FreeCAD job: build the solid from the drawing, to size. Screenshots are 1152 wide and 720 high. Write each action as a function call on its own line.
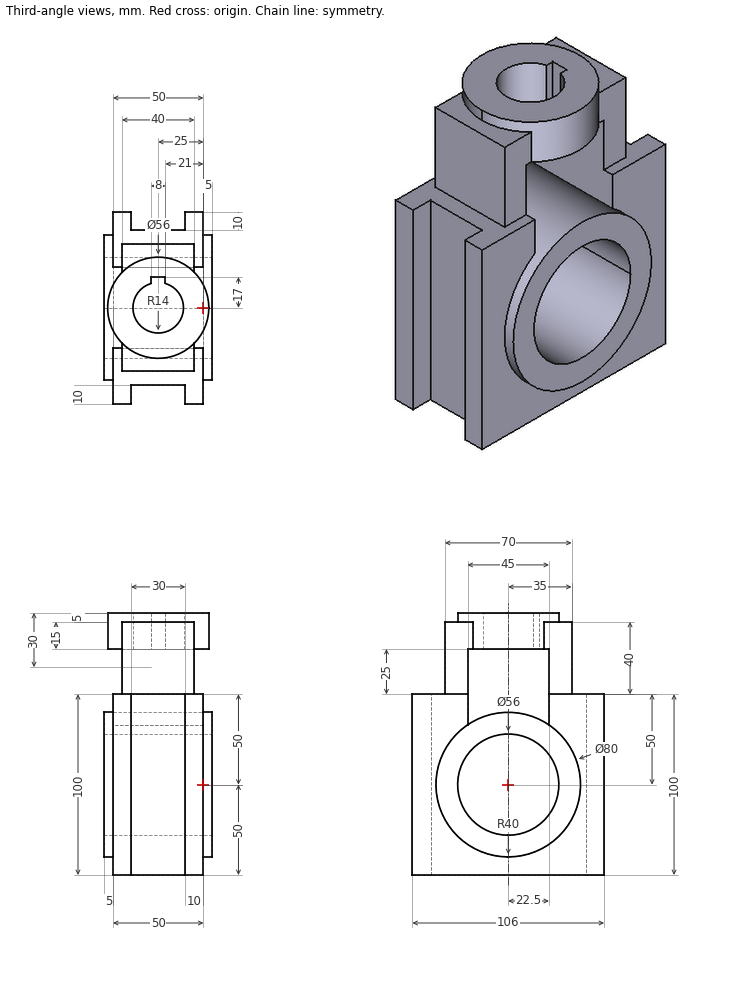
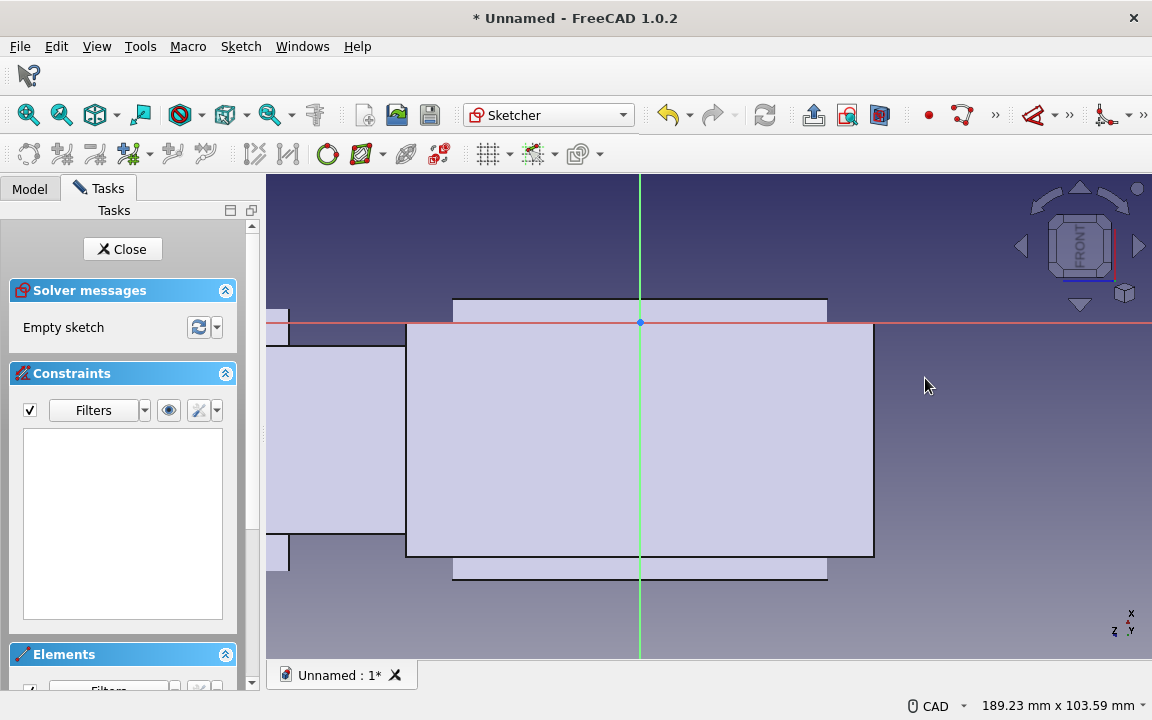
key(g)
key(r)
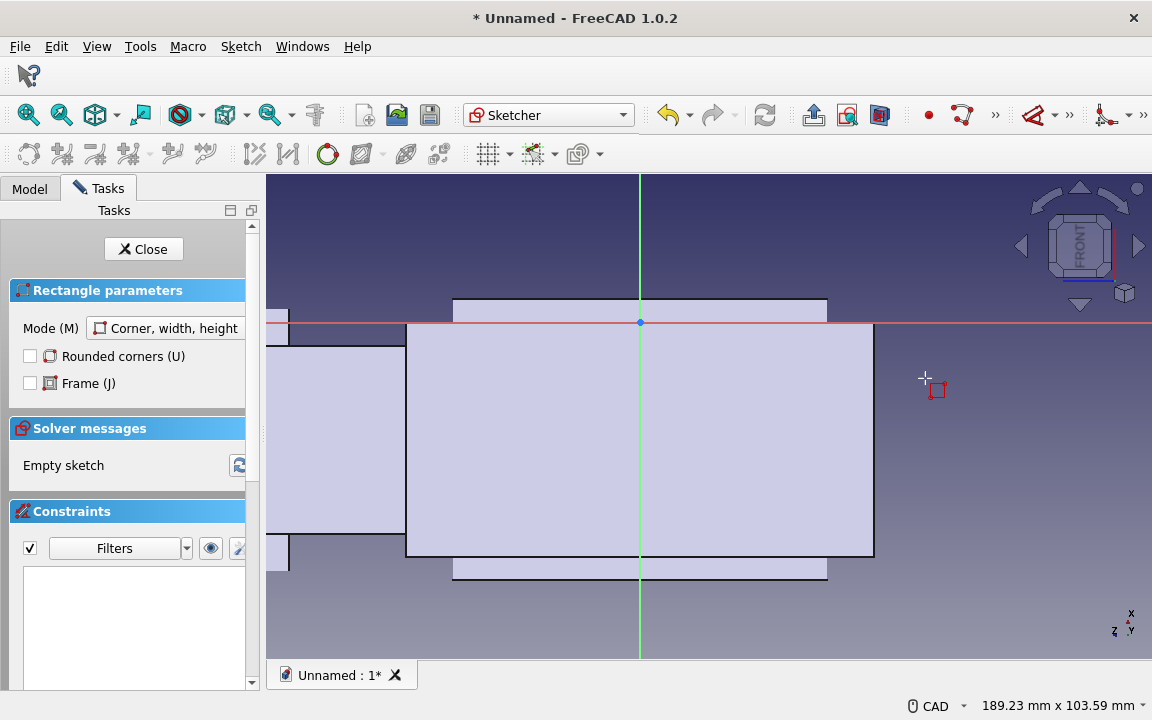
click(406, 370)
move(874, 510)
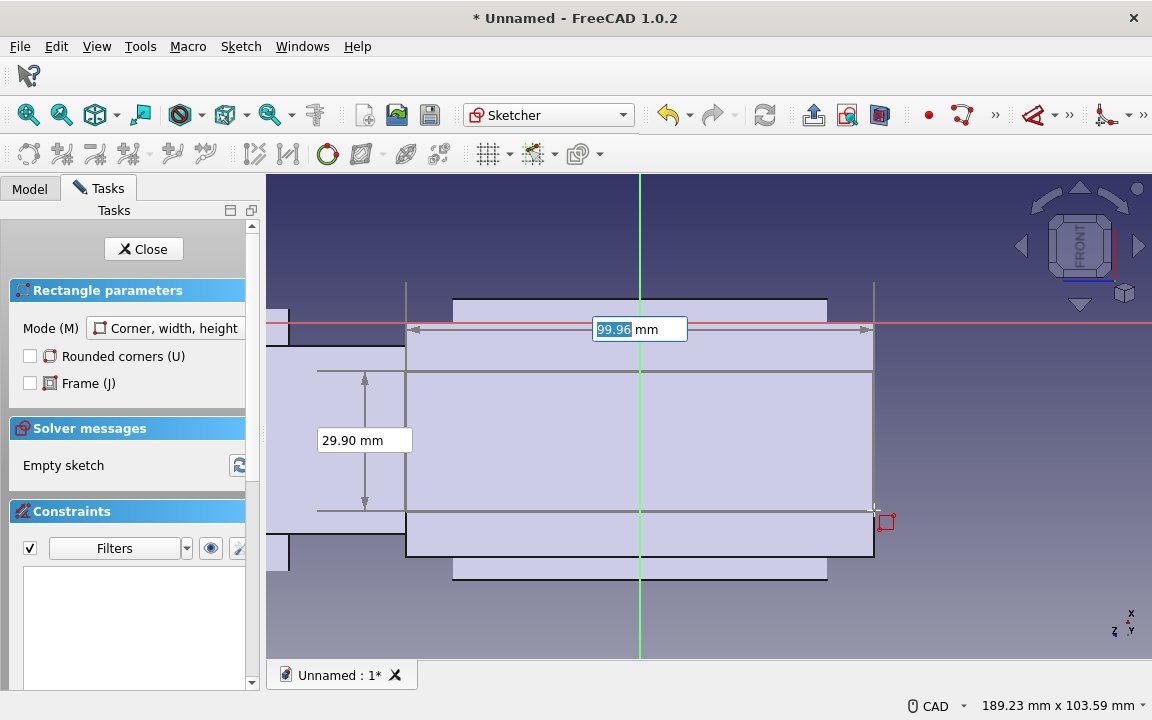
text(100)
key(Tab)
text(30)
key(Return)
key(Escape)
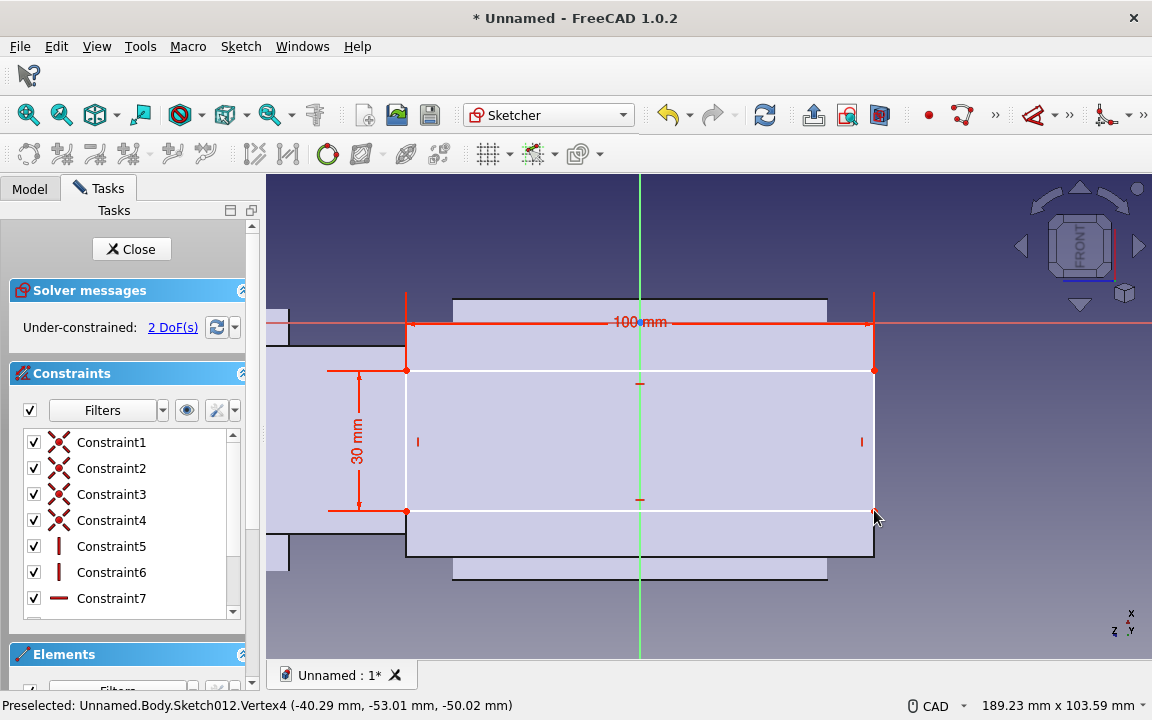
key(d)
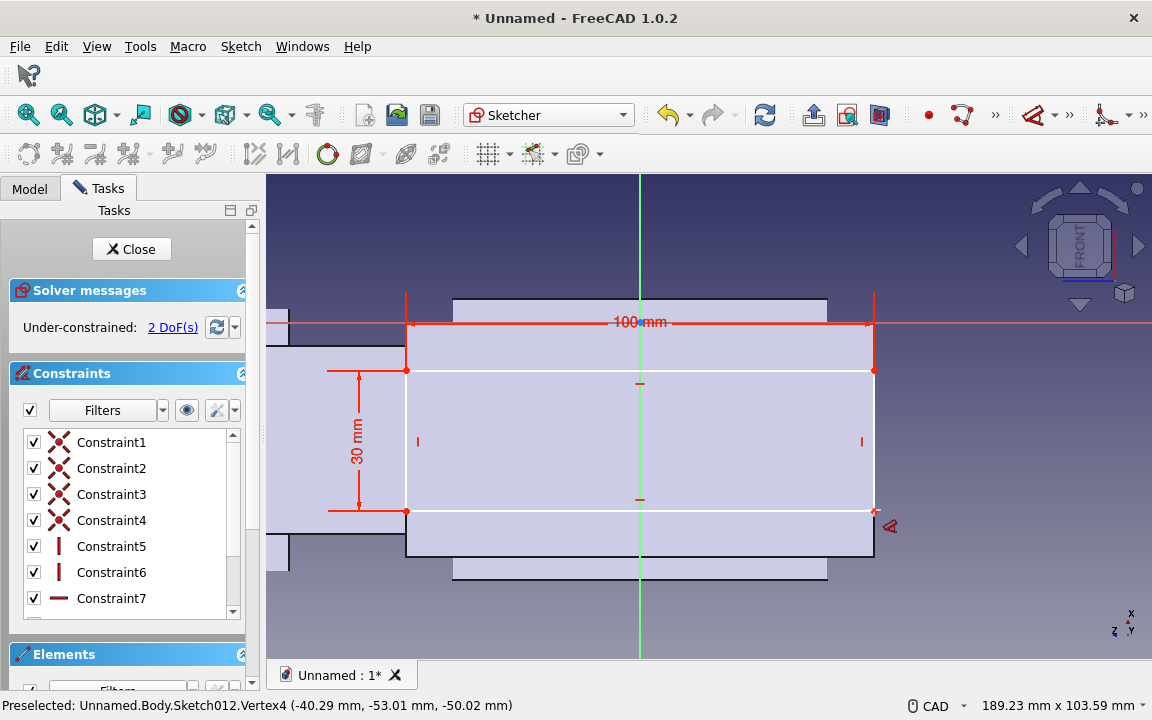
click(406, 371)
click(523, 289)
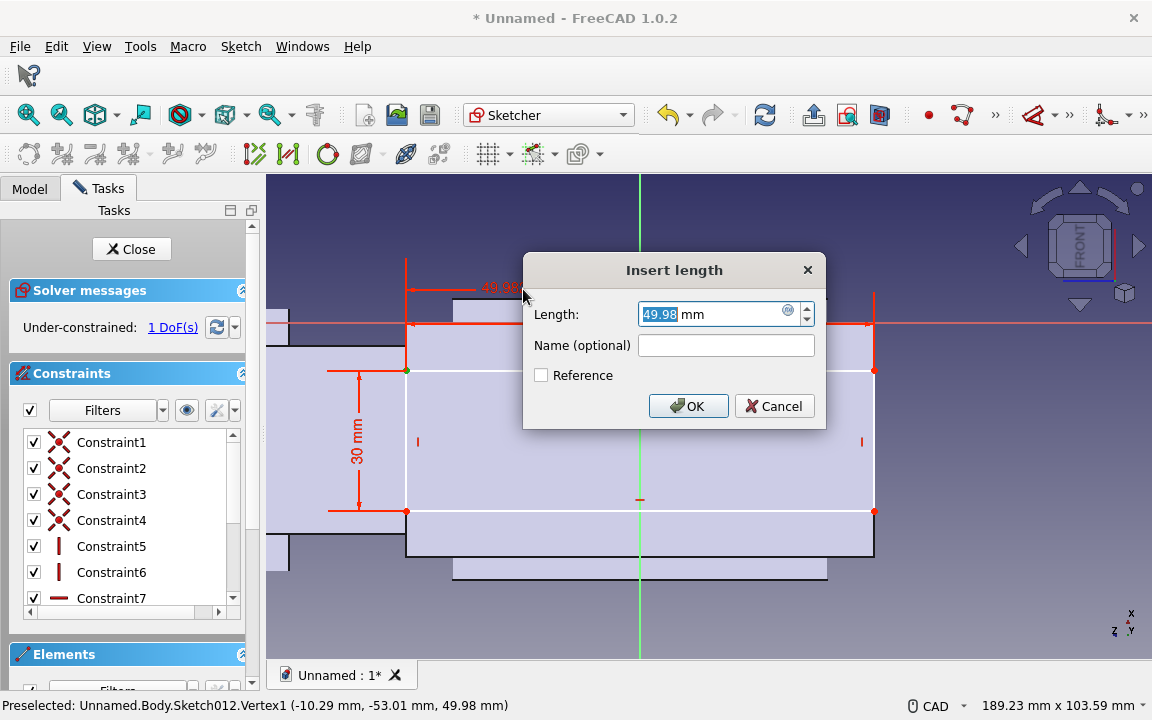
text(50)
key(Return)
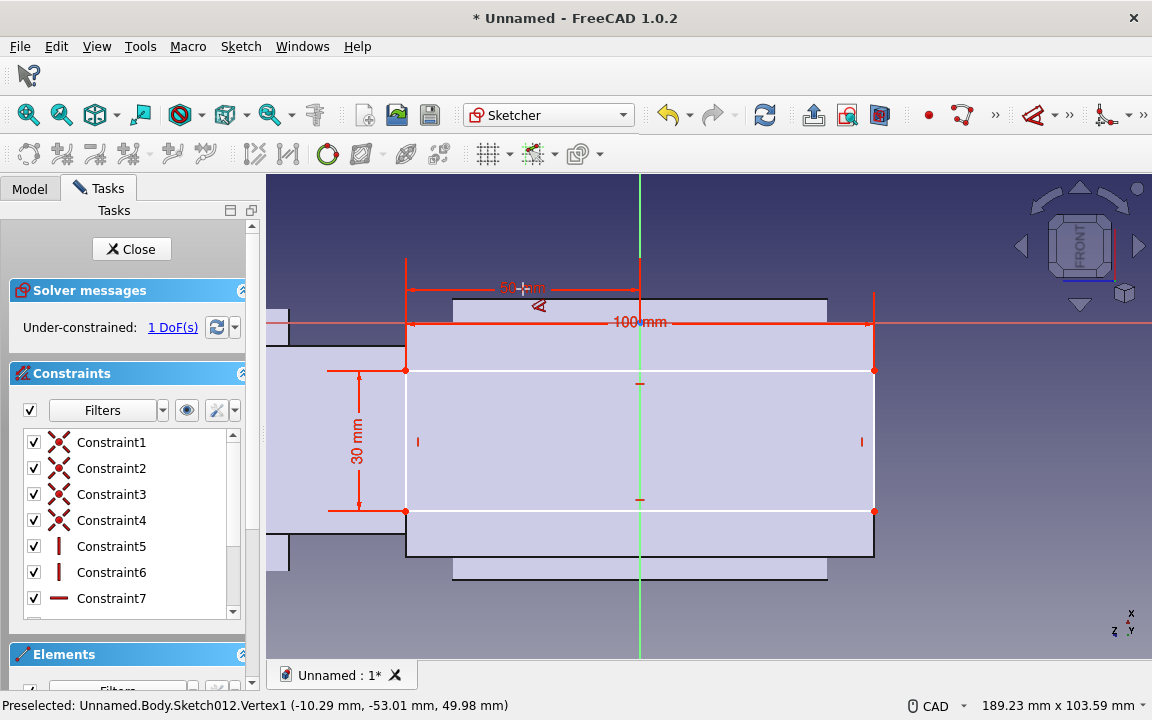
click(406, 371)
click(372, 347)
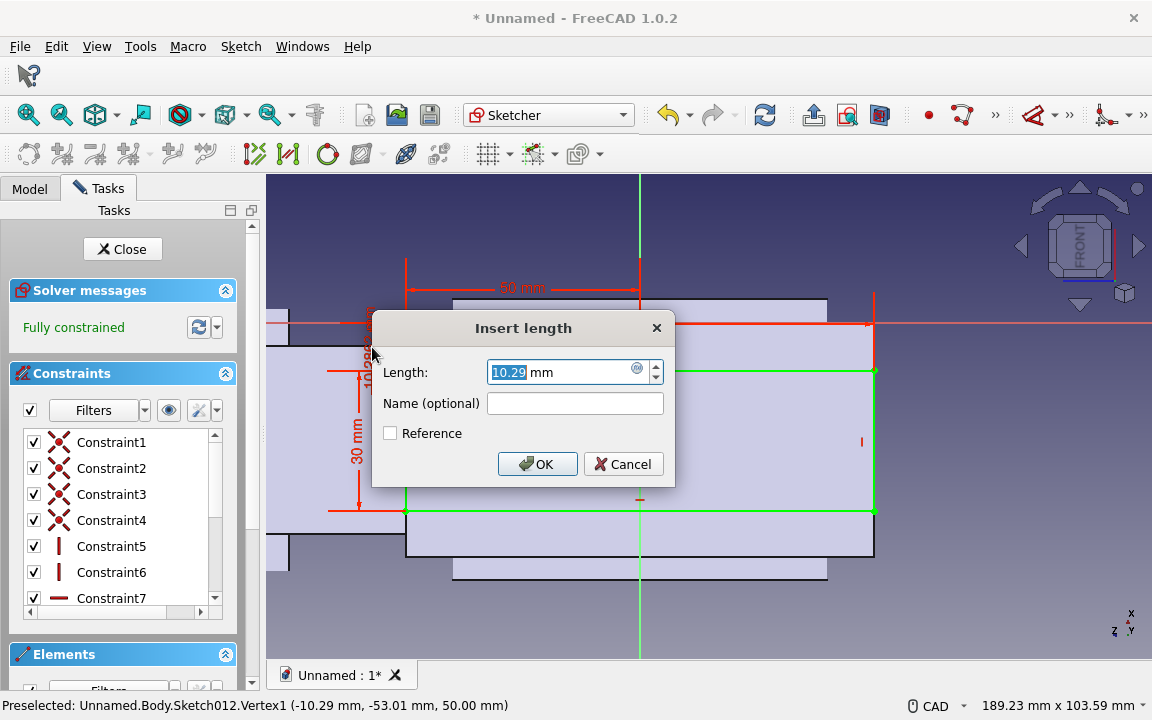
text(10)
key(Return)
key(Escape)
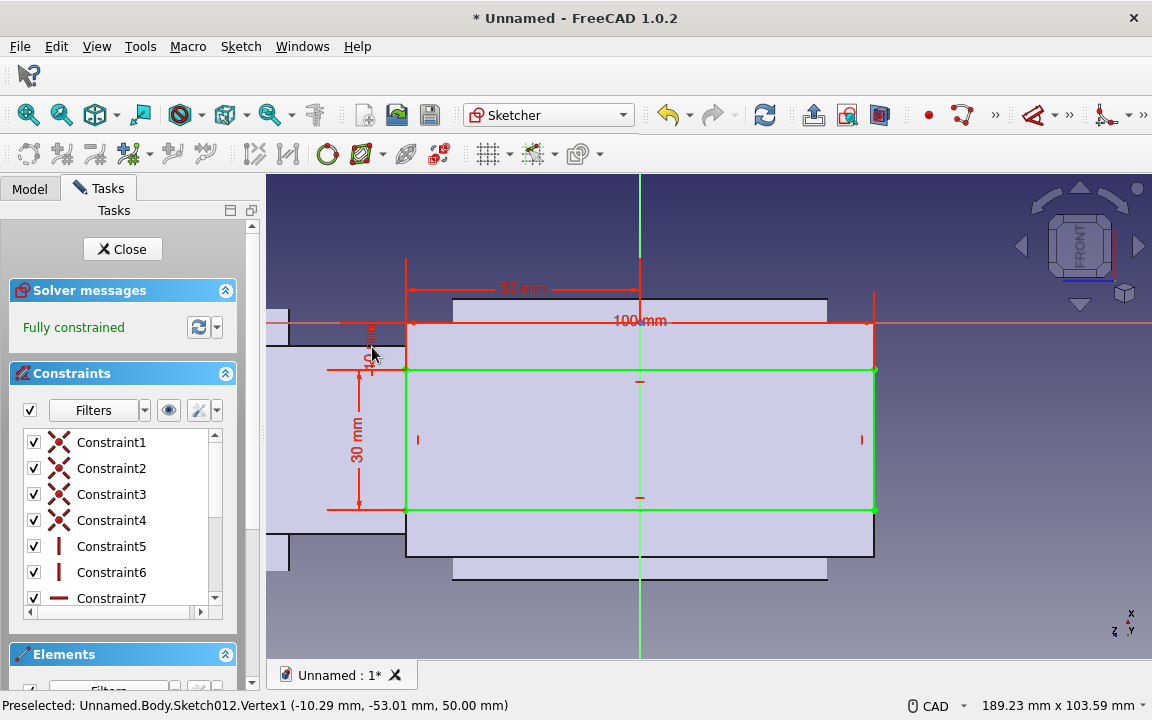
click(123, 249)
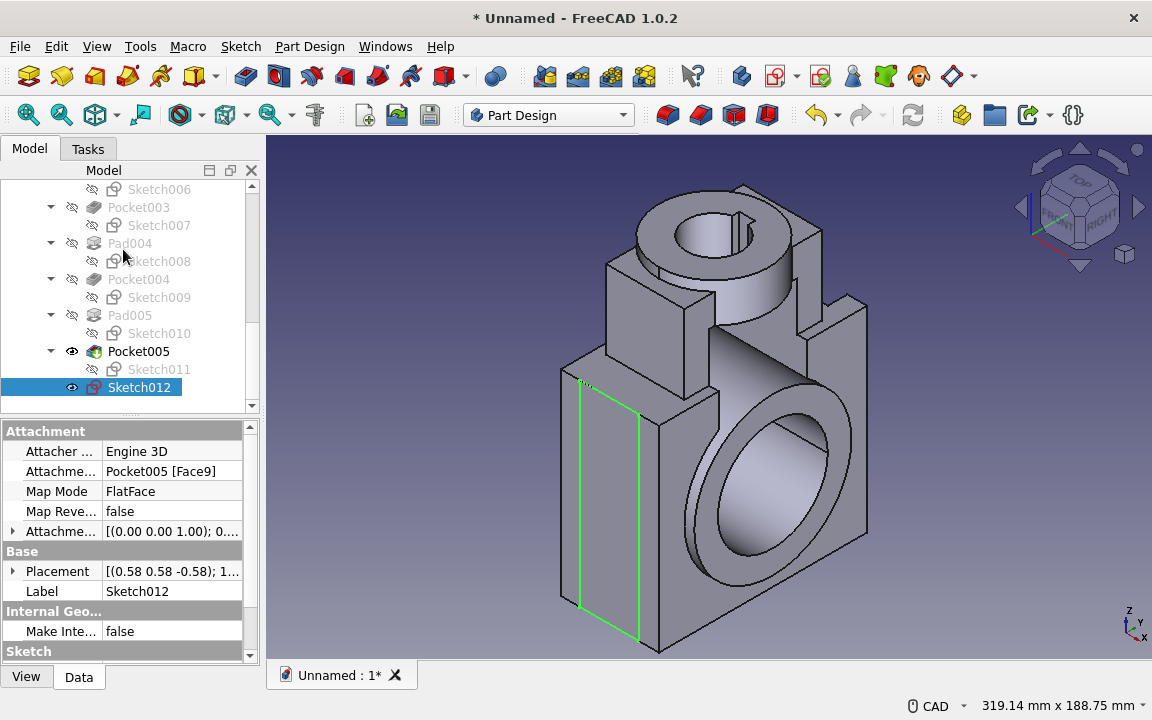
click(246, 76)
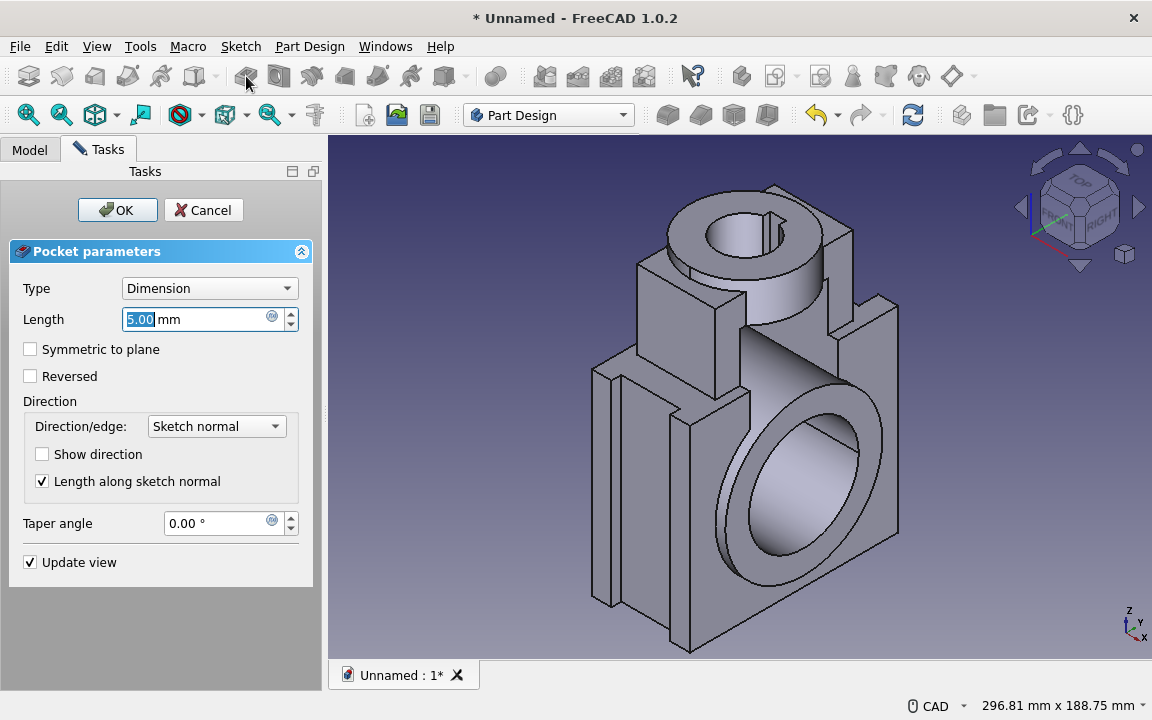
text(10)
key(Tab)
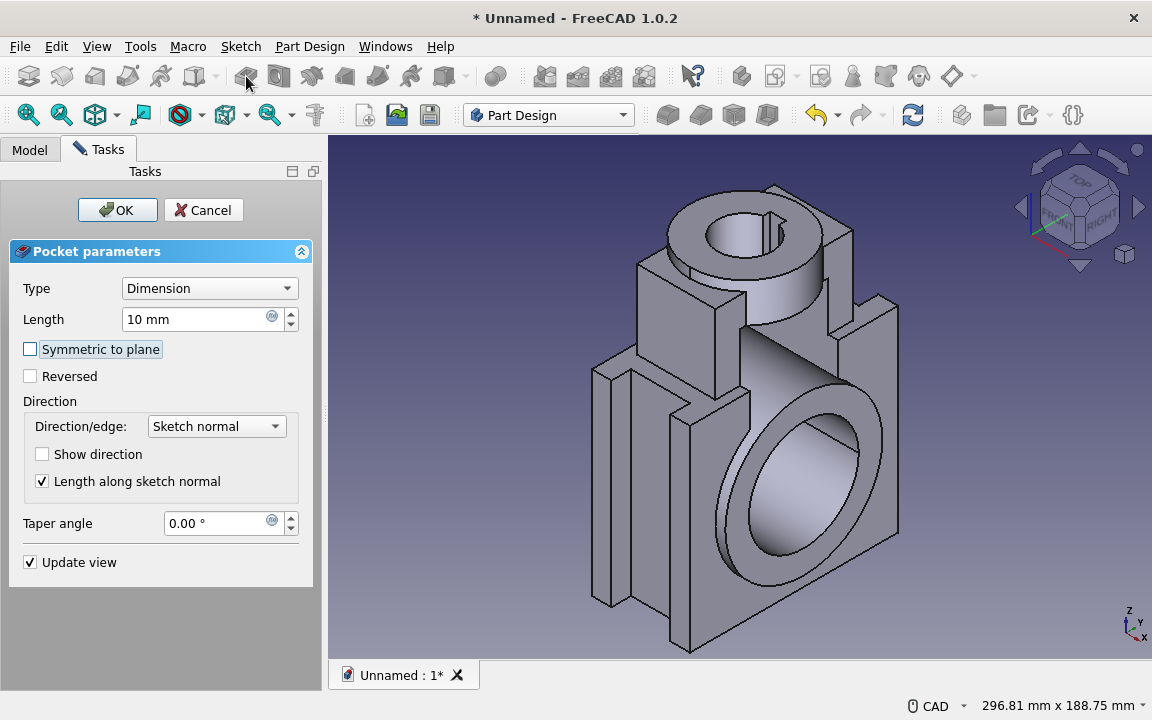
click(118, 210)